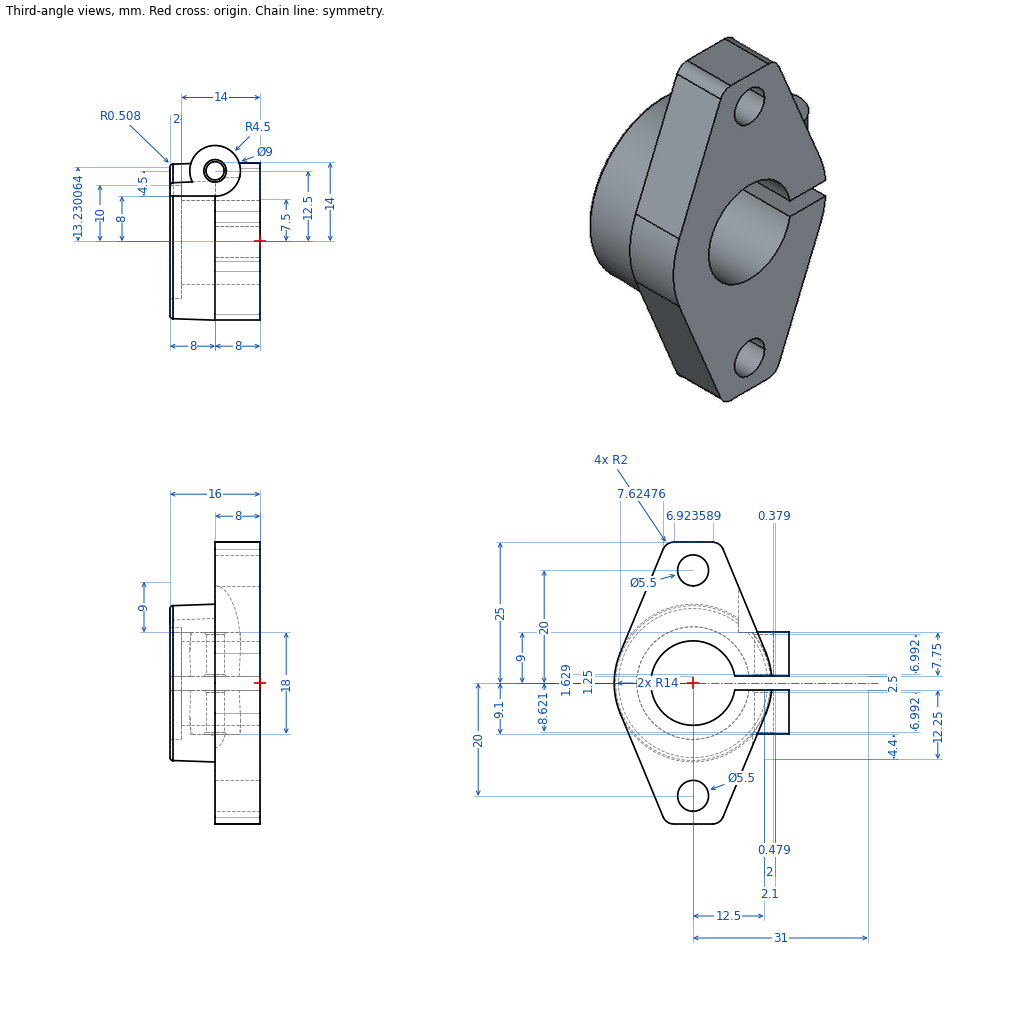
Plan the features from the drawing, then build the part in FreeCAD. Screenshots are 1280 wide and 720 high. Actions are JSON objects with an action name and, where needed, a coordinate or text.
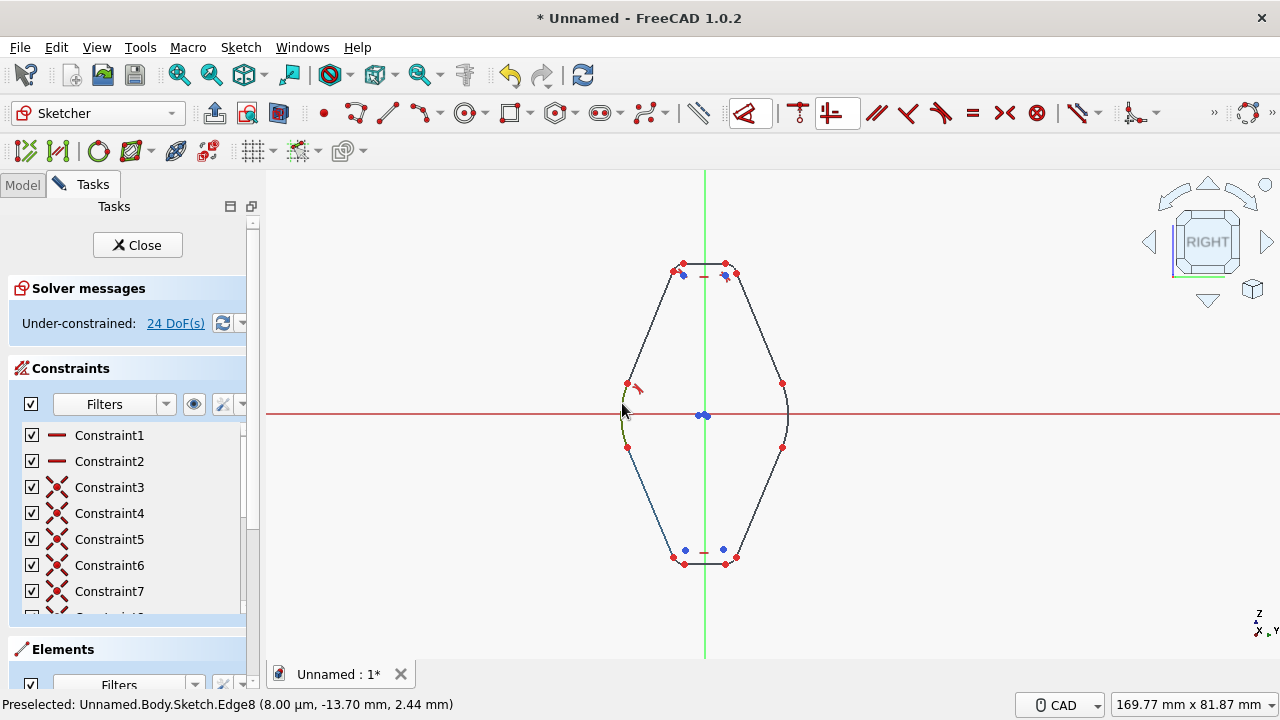
{"action": "left_click", "coordinate": [942, 114]}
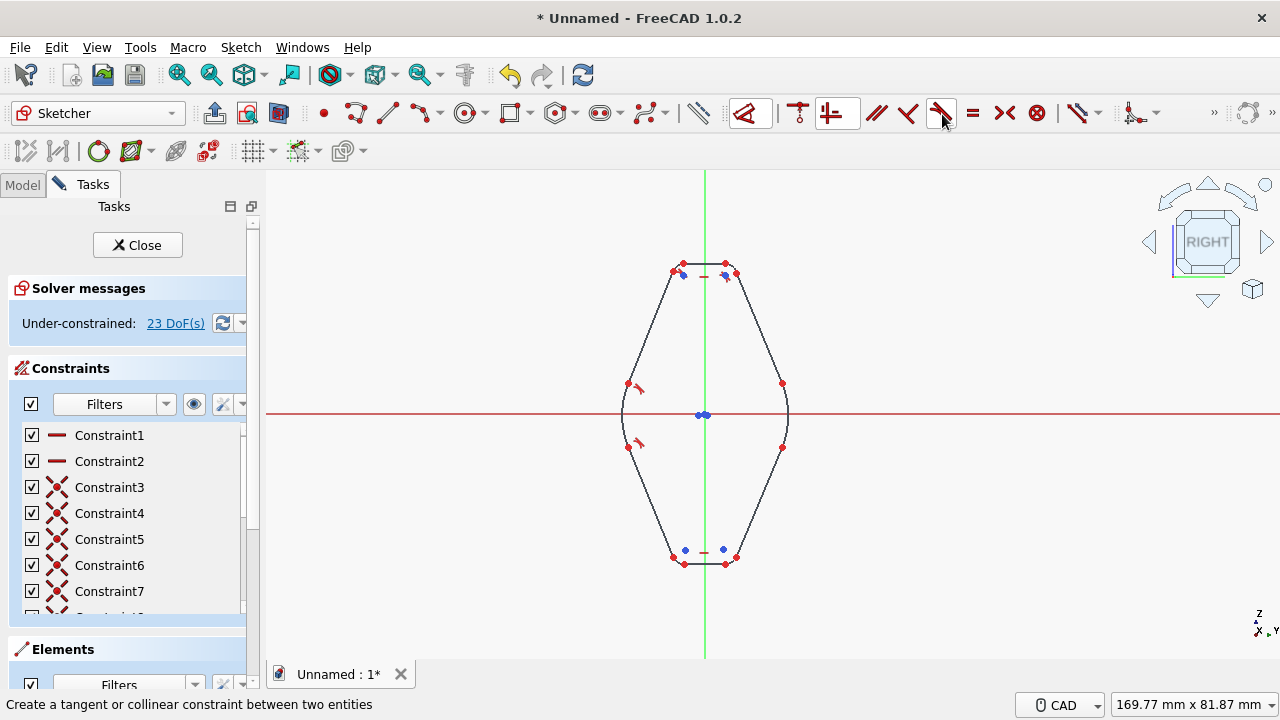
{"action": "left_click", "coordinate": [642, 480]}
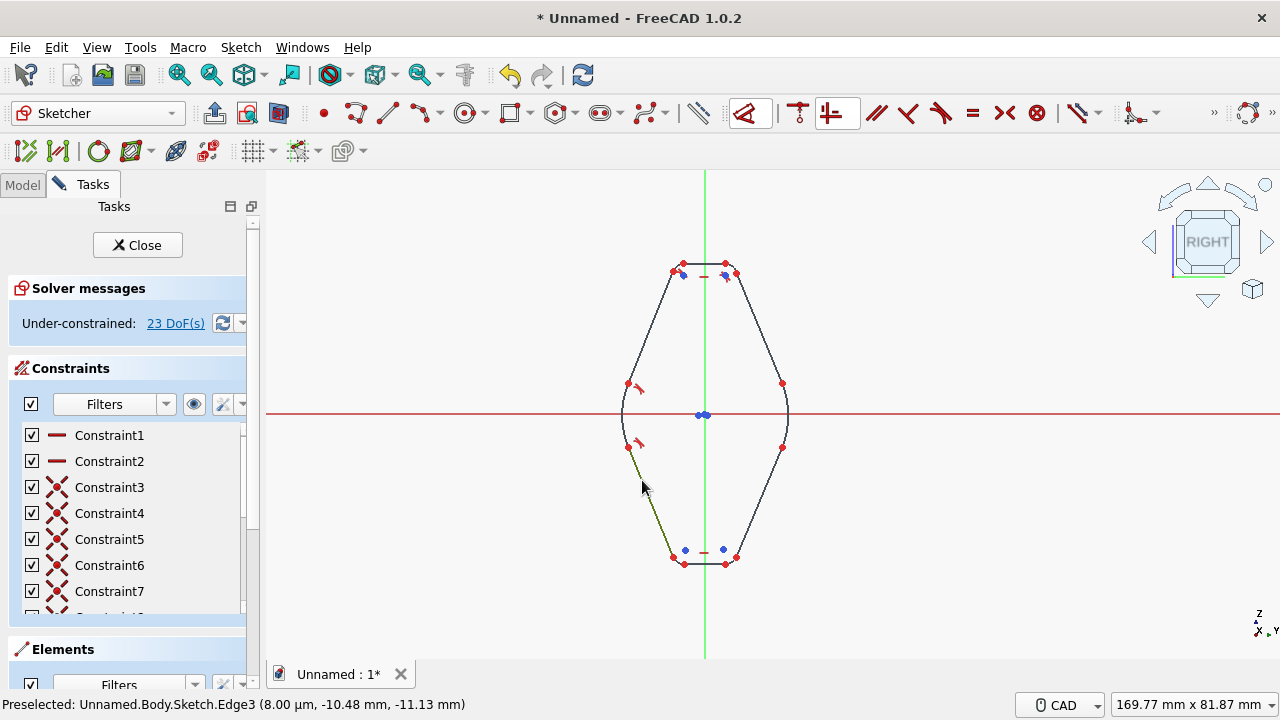
{"action": "scroll", "coordinate": [678, 562], "scroll_direction": "up", "scroll_amount": 4}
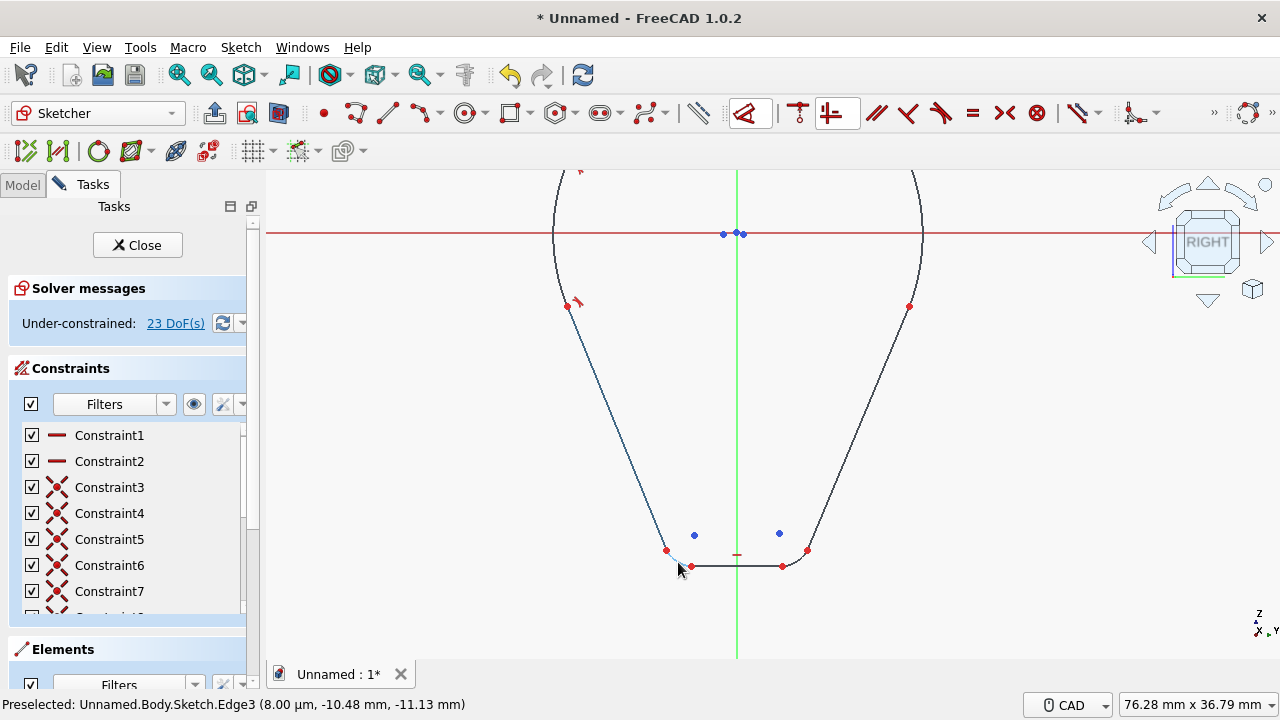
{"action": "left_click", "coordinate": [677, 562]}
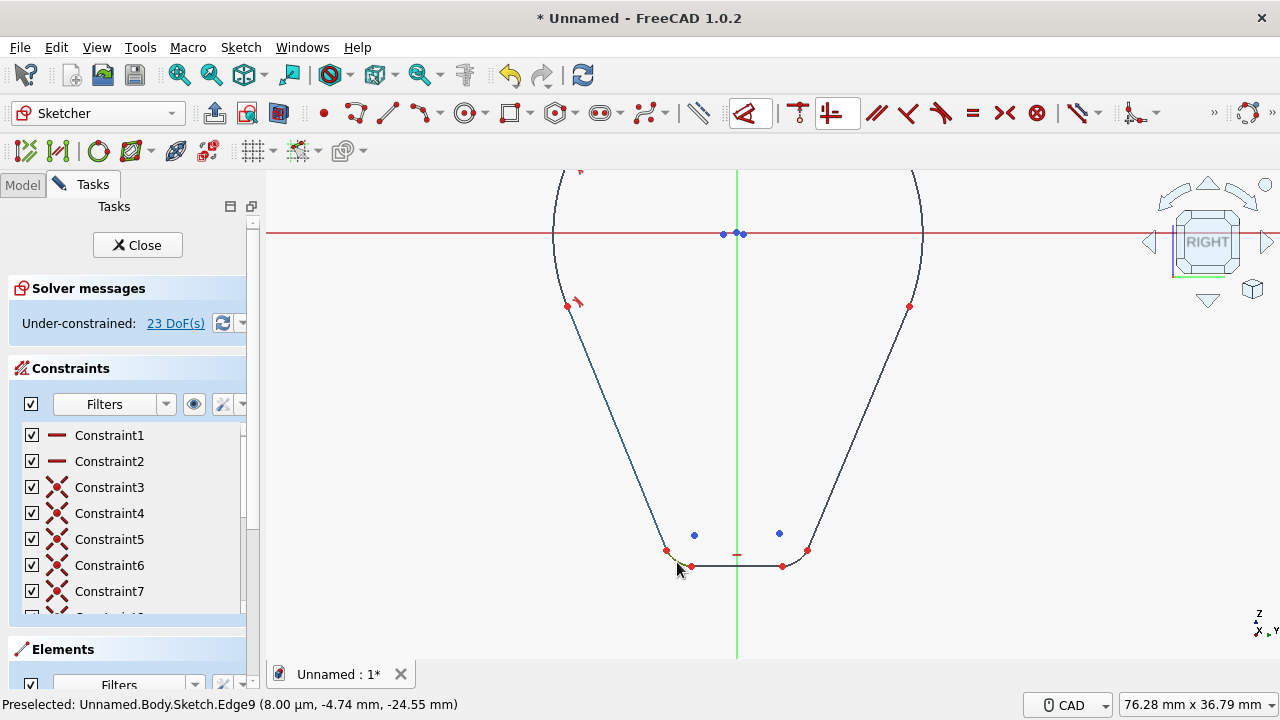
{"action": "key", "text": "t"}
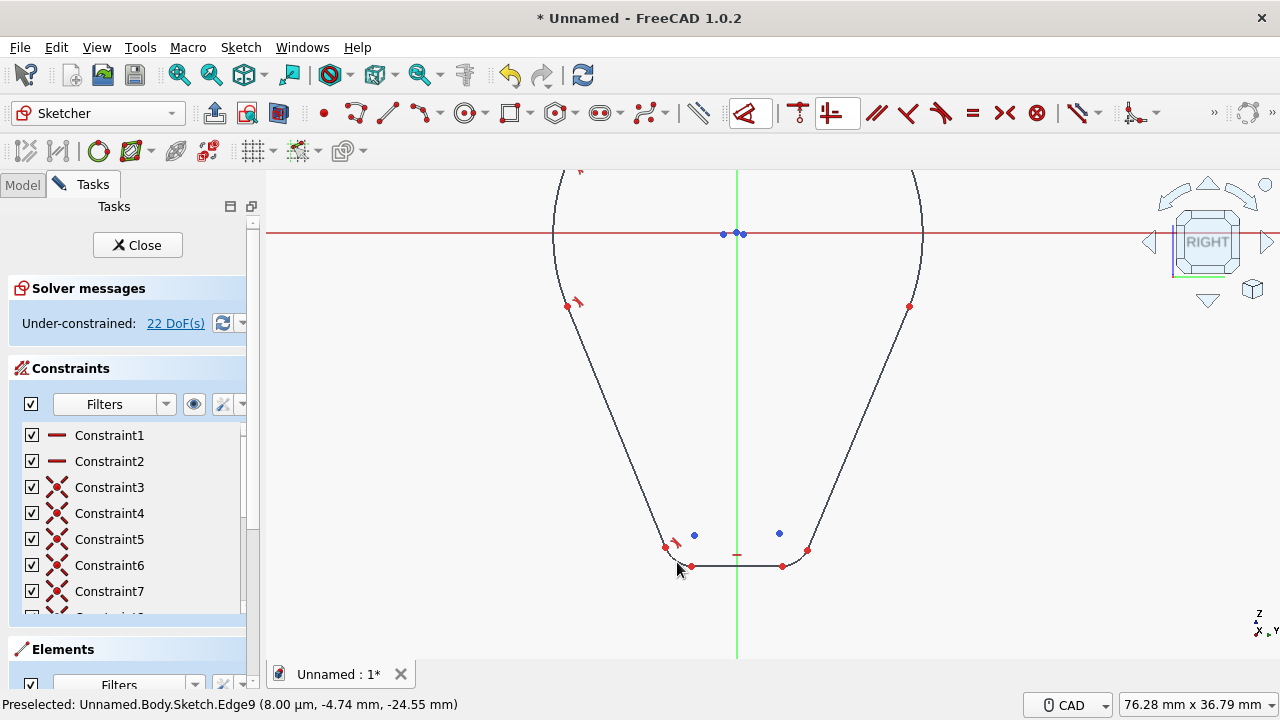
{"action": "left_click", "coordinate": [719, 566]}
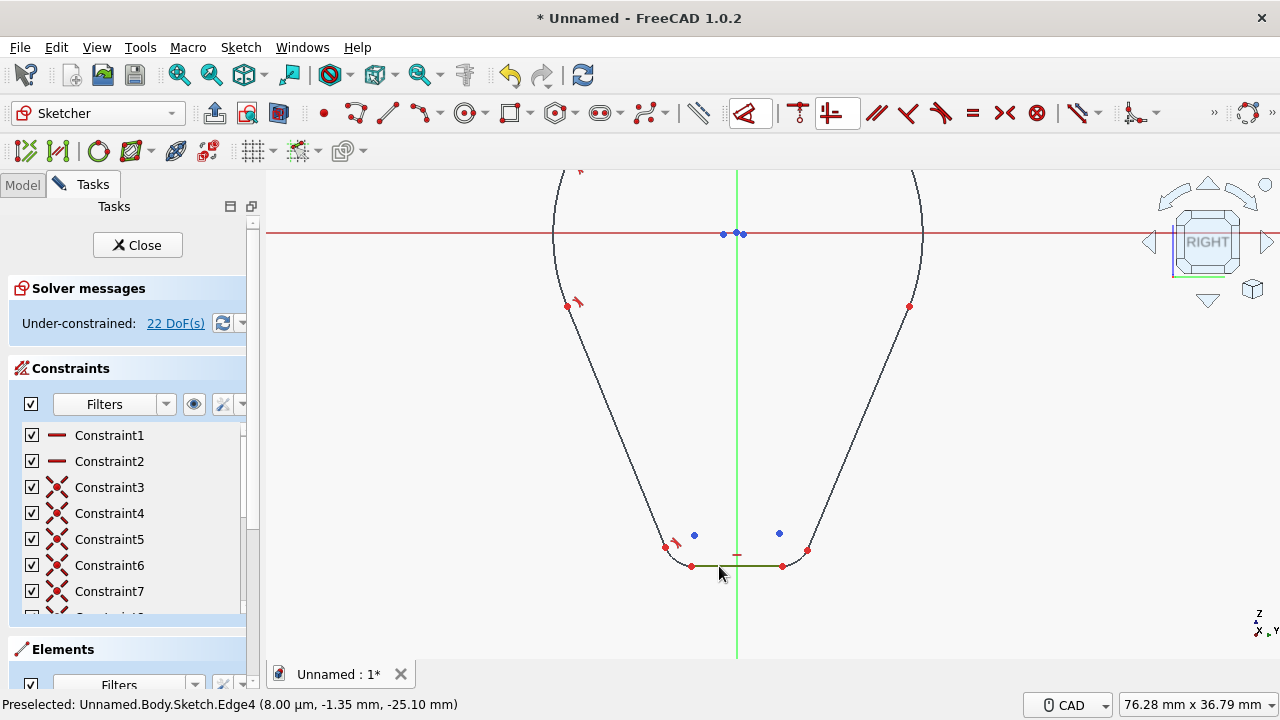
{"action": "scroll", "coordinate": [671, 556], "scroll_direction": "up", "scroll_amount": 2}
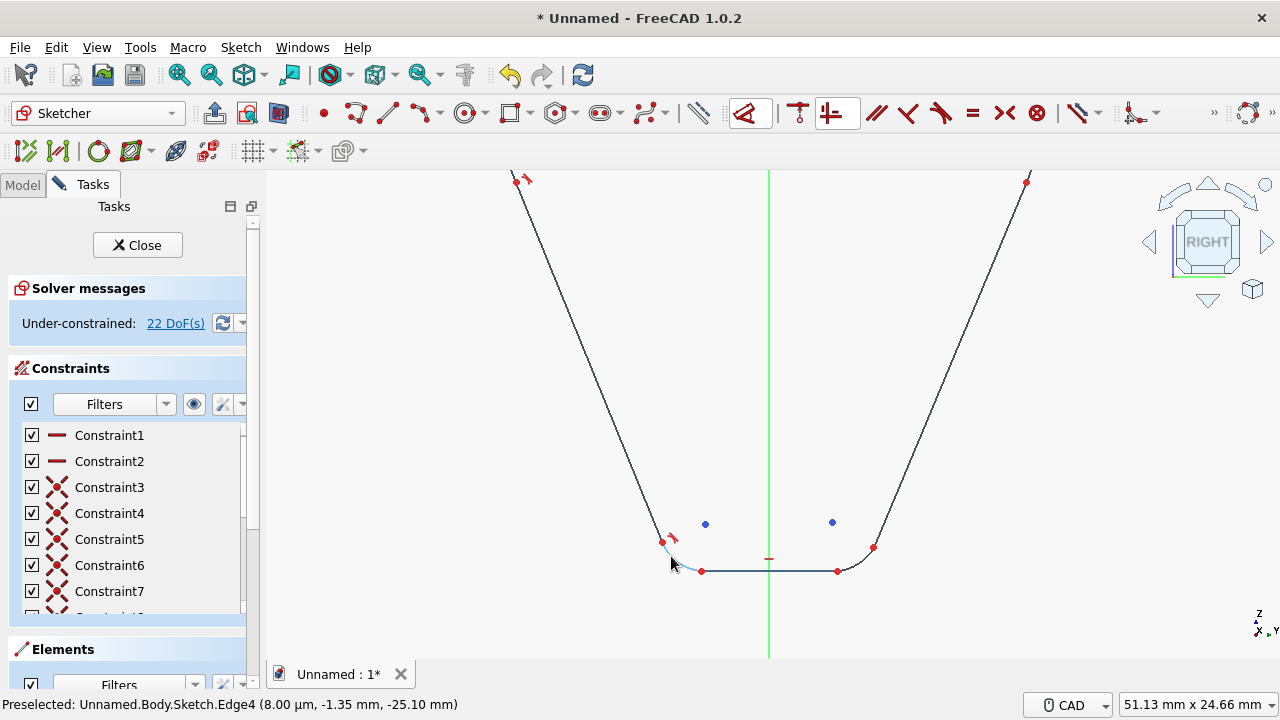
{"action": "left_click", "coordinate": [670, 555]}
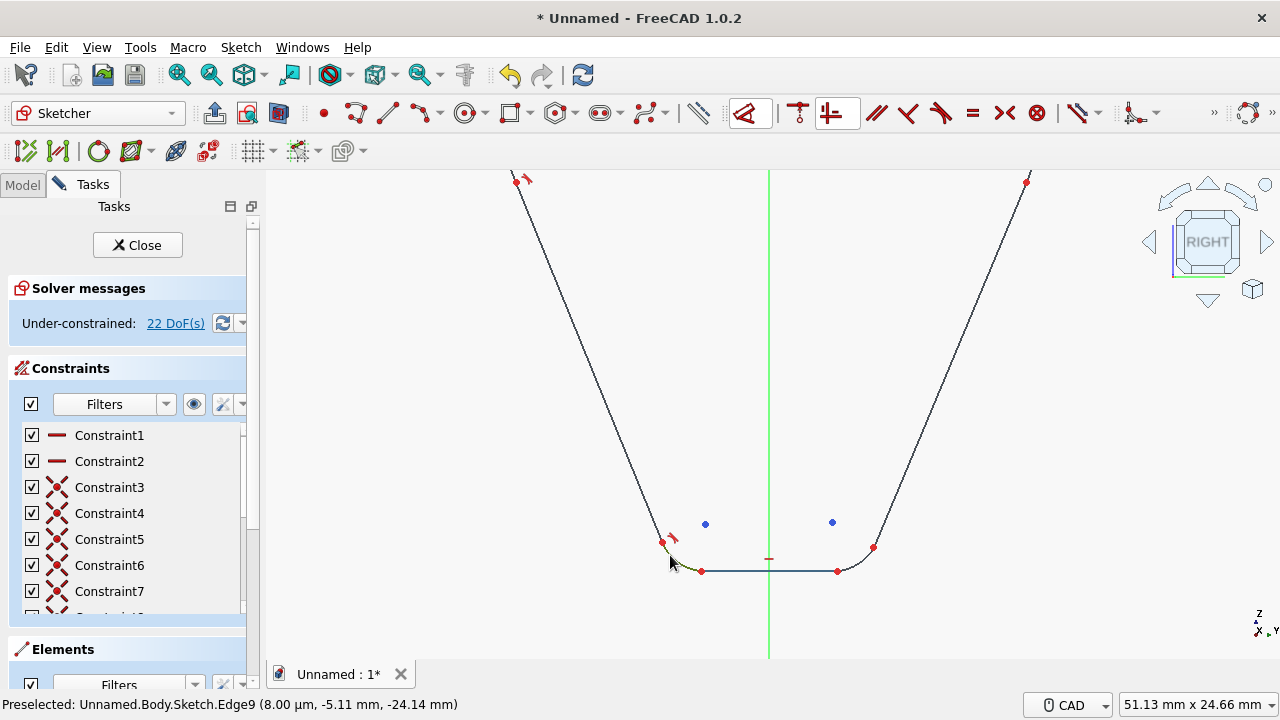
{"action": "left_click", "coordinate": [942, 114]}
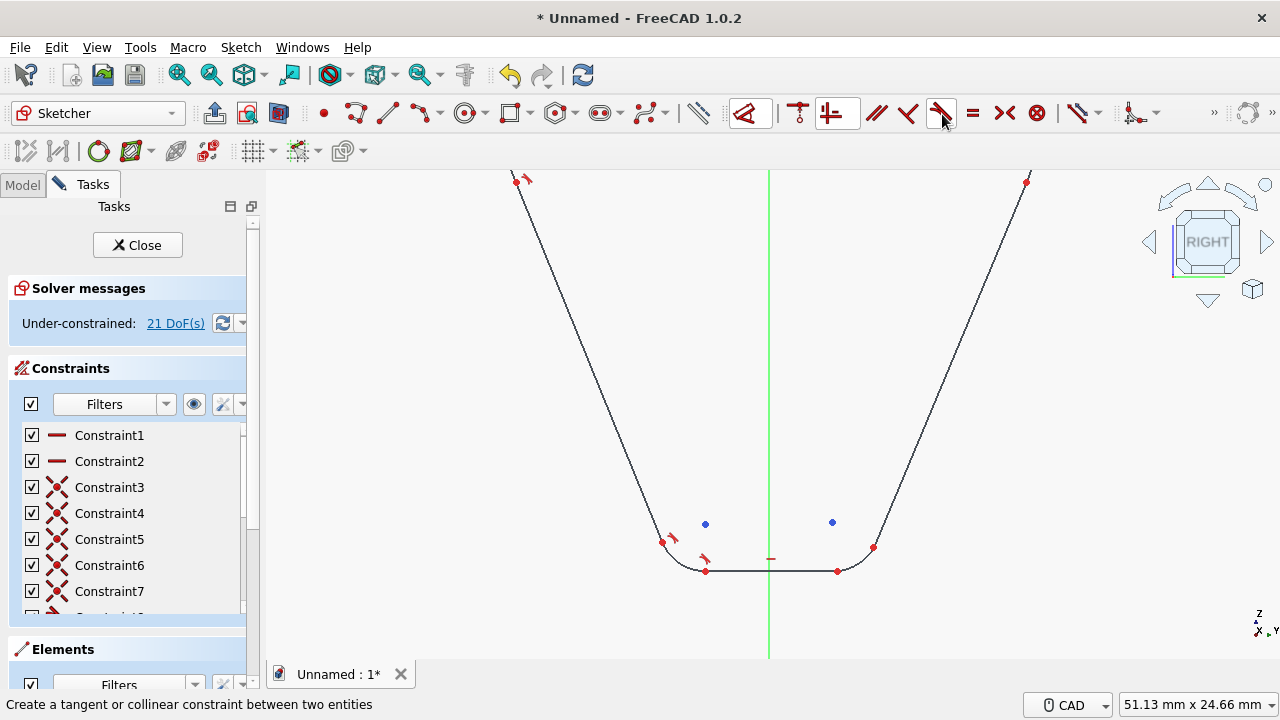
{"action": "left_click", "coordinate": [745, 571]}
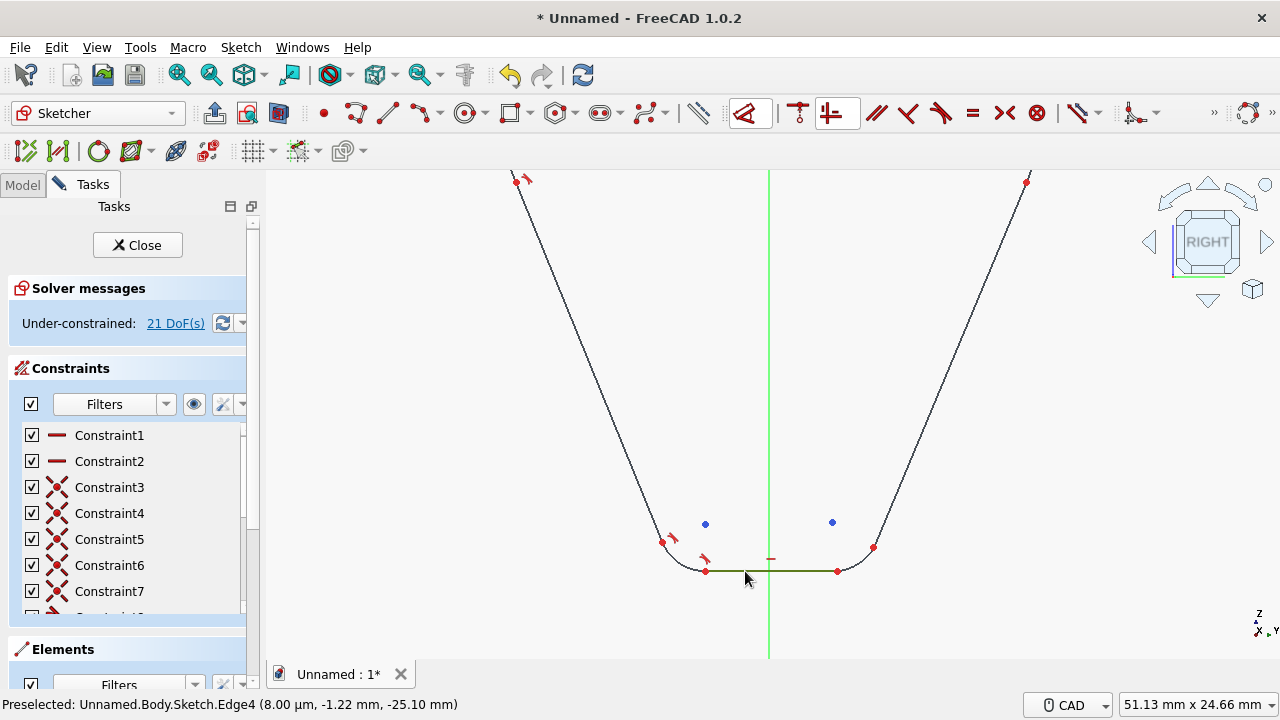
{"action": "left_click", "coordinate": [850, 568]}